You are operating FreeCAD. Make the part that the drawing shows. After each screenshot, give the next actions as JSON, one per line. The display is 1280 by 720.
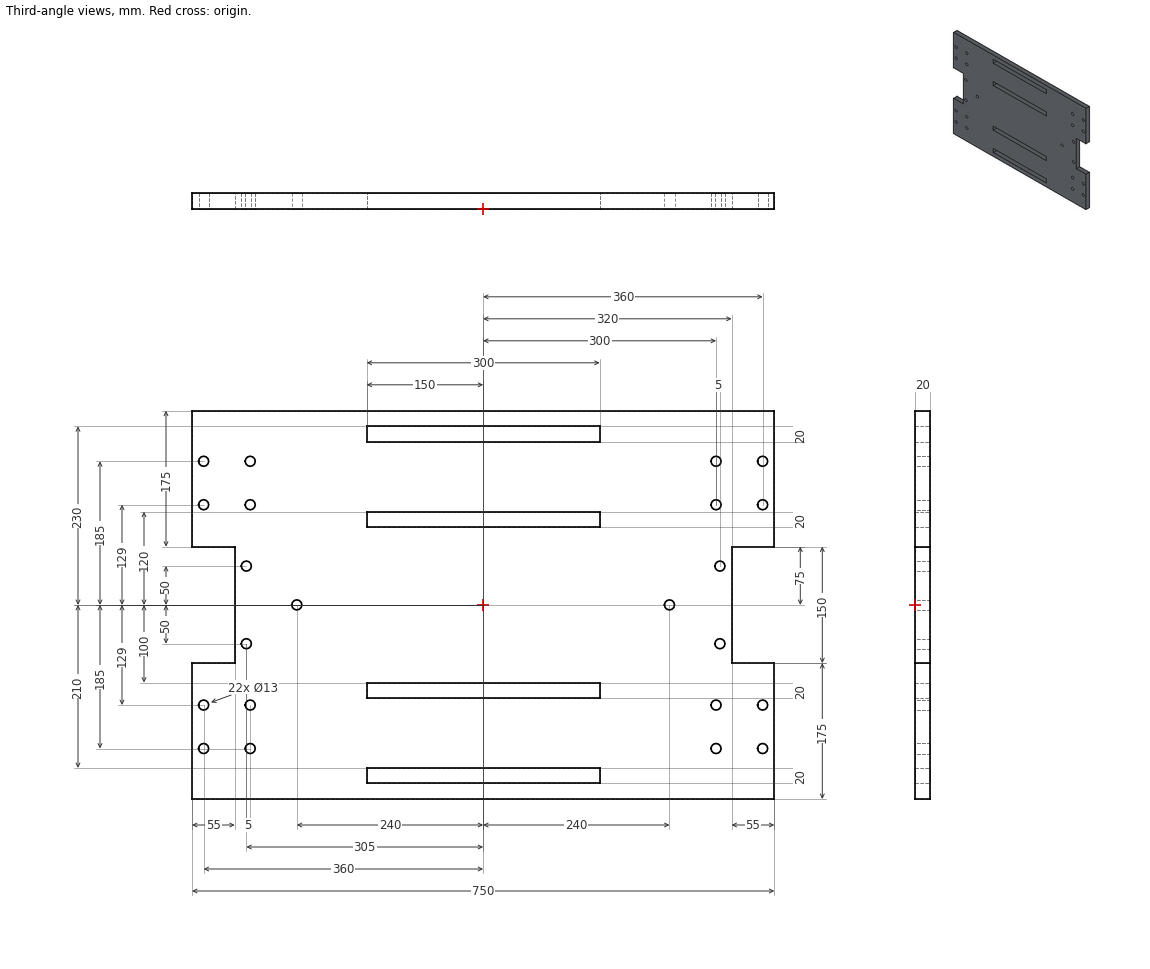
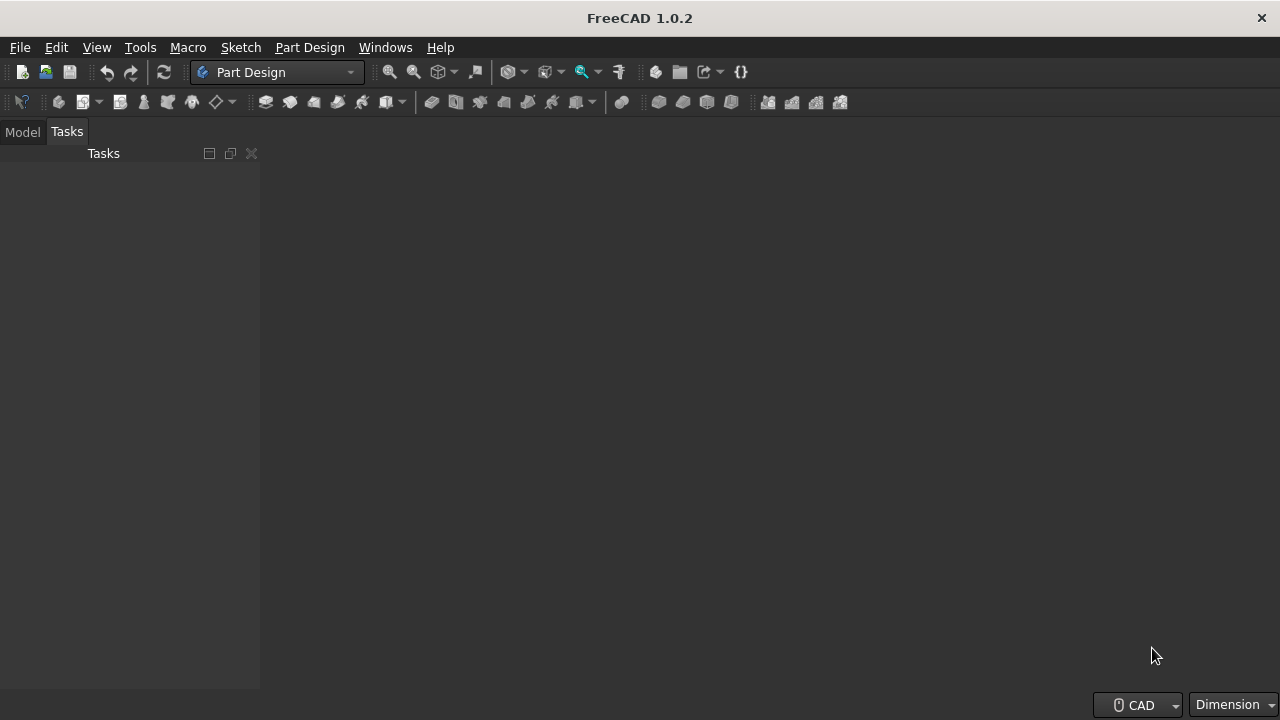
{"action": "left_click", "coordinate": [22, 72]}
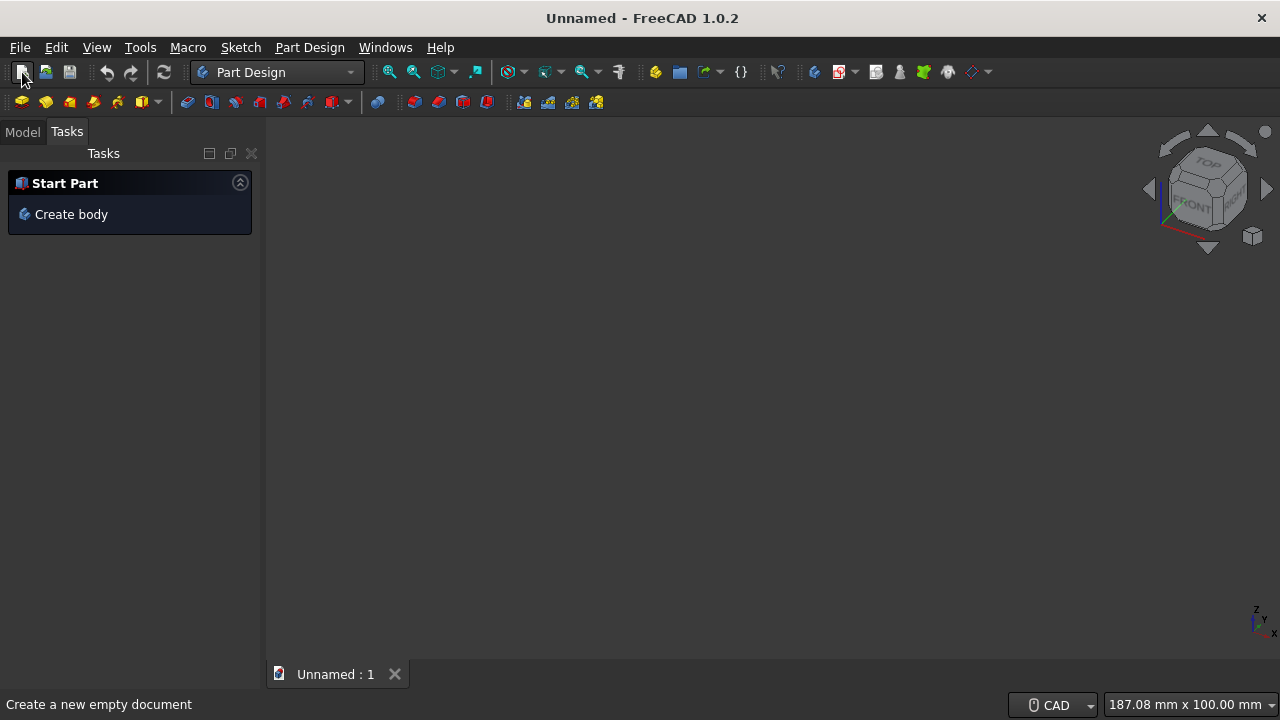
{"action": "left_click", "coordinate": [840, 72]}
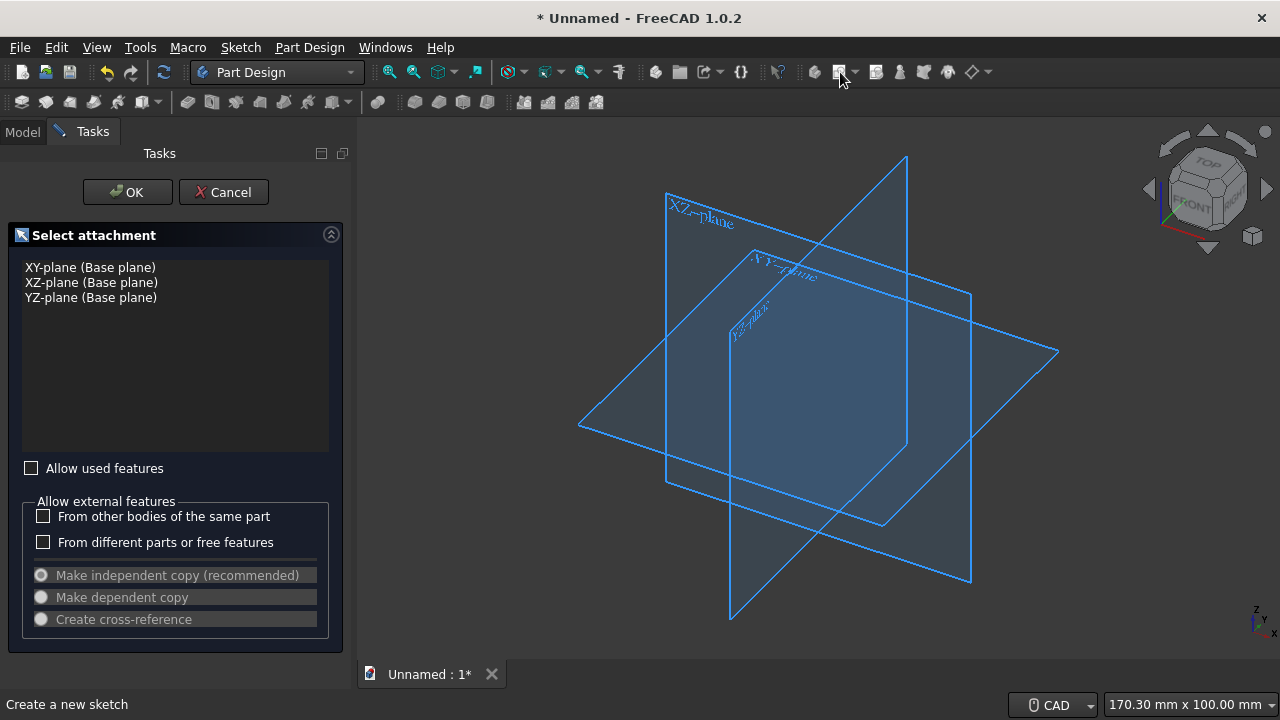
{"action": "left_click", "coordinate": [82, 282]}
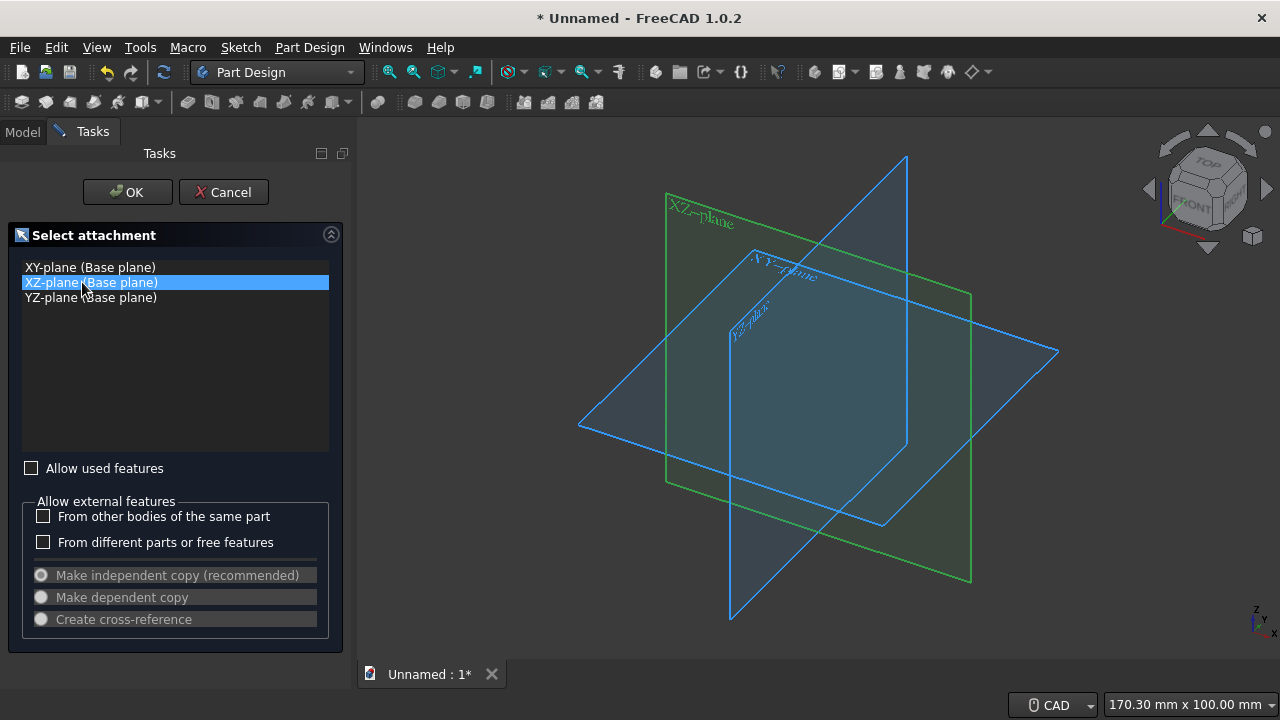
{"action": "left_click", "coordinate": [128, 192]}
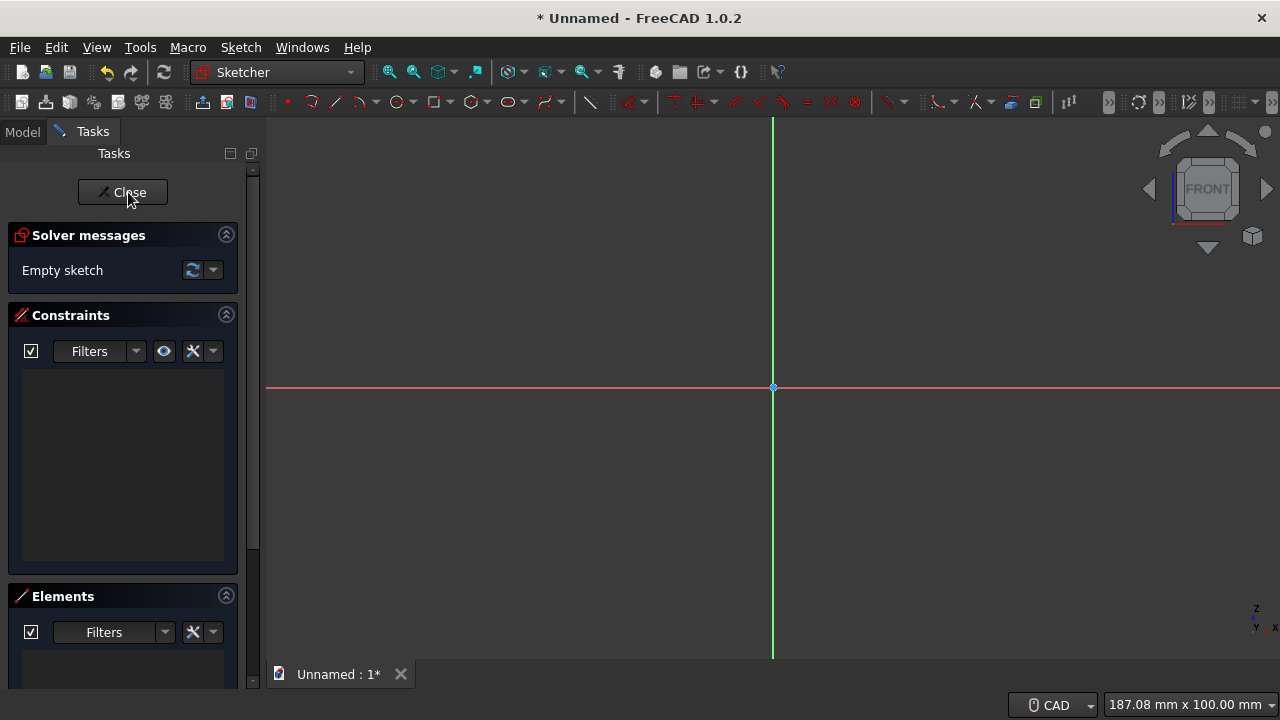
{"action": "scroll", "coordinate": [694, 388], "scroll_direction": "down", "scroll_amount": 10}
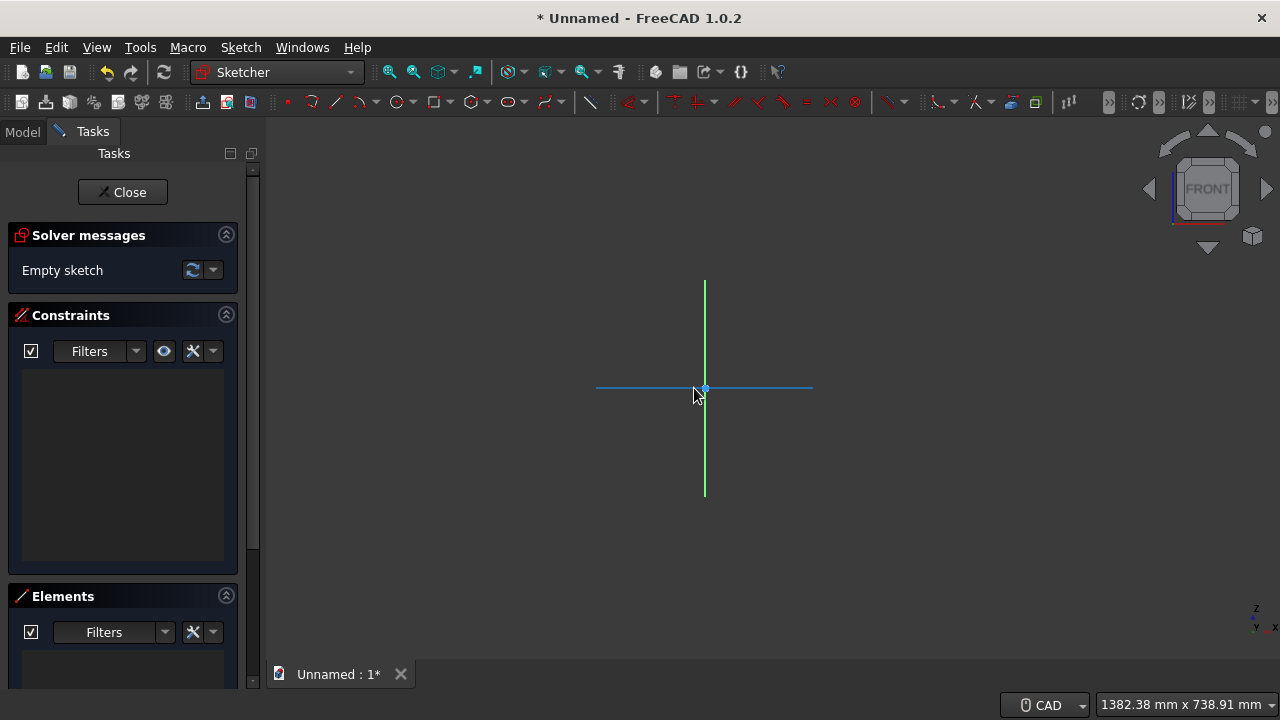
{"action": "left_click", "coordinate": [312, 102]}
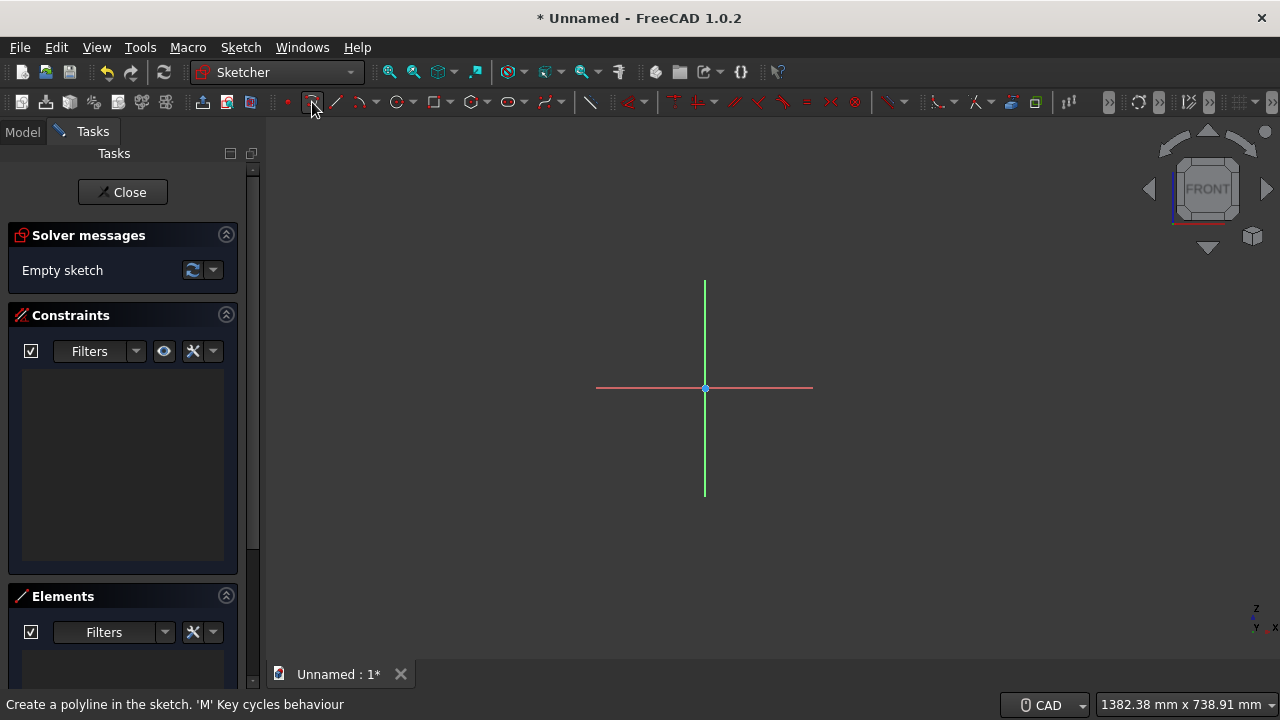
{"action": "left_click", "coordinate": [940, 333]}
{"action": "left_click", "coordinate": [940, 443]}
{"action": "left_click", "coordinate": [980, 443]}
{"action": "left_click", "coordinate": [980, 572]}
{"action": "left_click", "coordinate": [430, 572]}
{"action": "left_click", "coordinate": [430, 443]}
{"action": "left_click", "coordinate": [470, 443]}
{"action": "left_click", "coordinate": [470, 333]}
{"action": "left_click", "coordinate": [430, 333]}
{"action": "left_click", "coordinate": [430, 205]}
{"action": "left_click", "coordinate": [980, 205]}
{"action": "left_click", "coordinate": [980, 333]}
{"action": "left_click", "coordinate": [940, 334]}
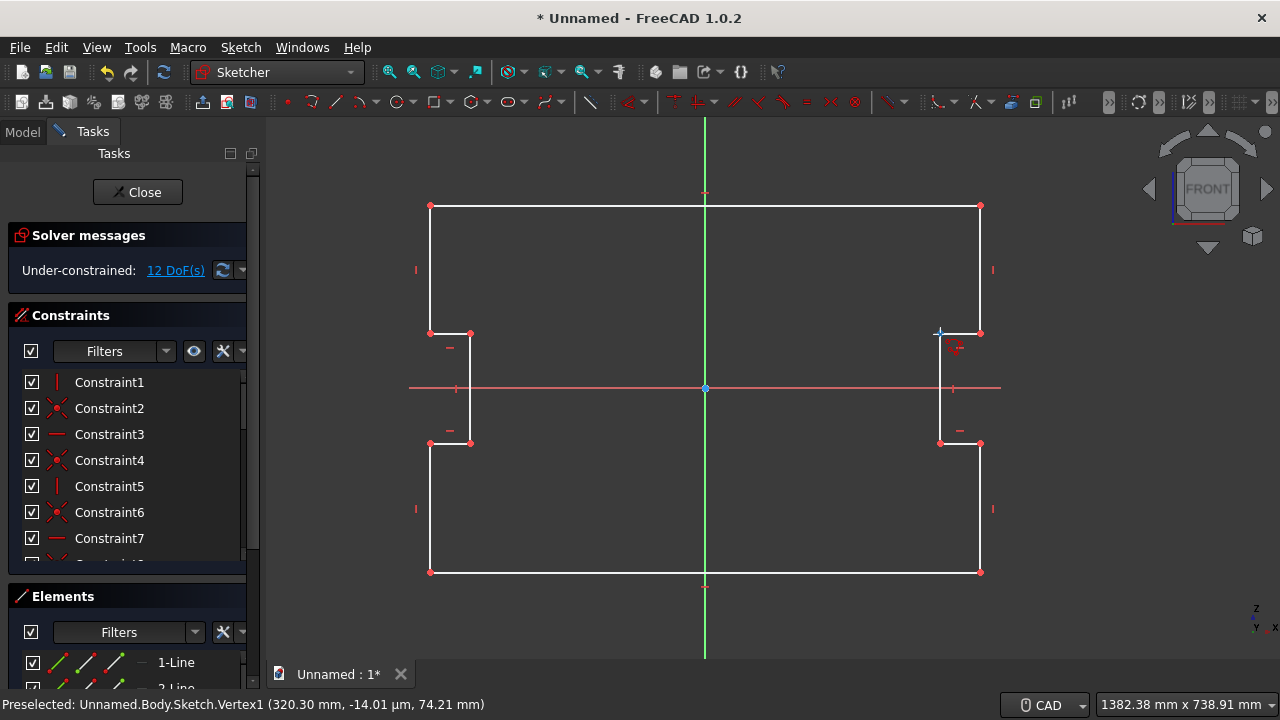
{"action": "left_click", "coordinate": [434, 102]}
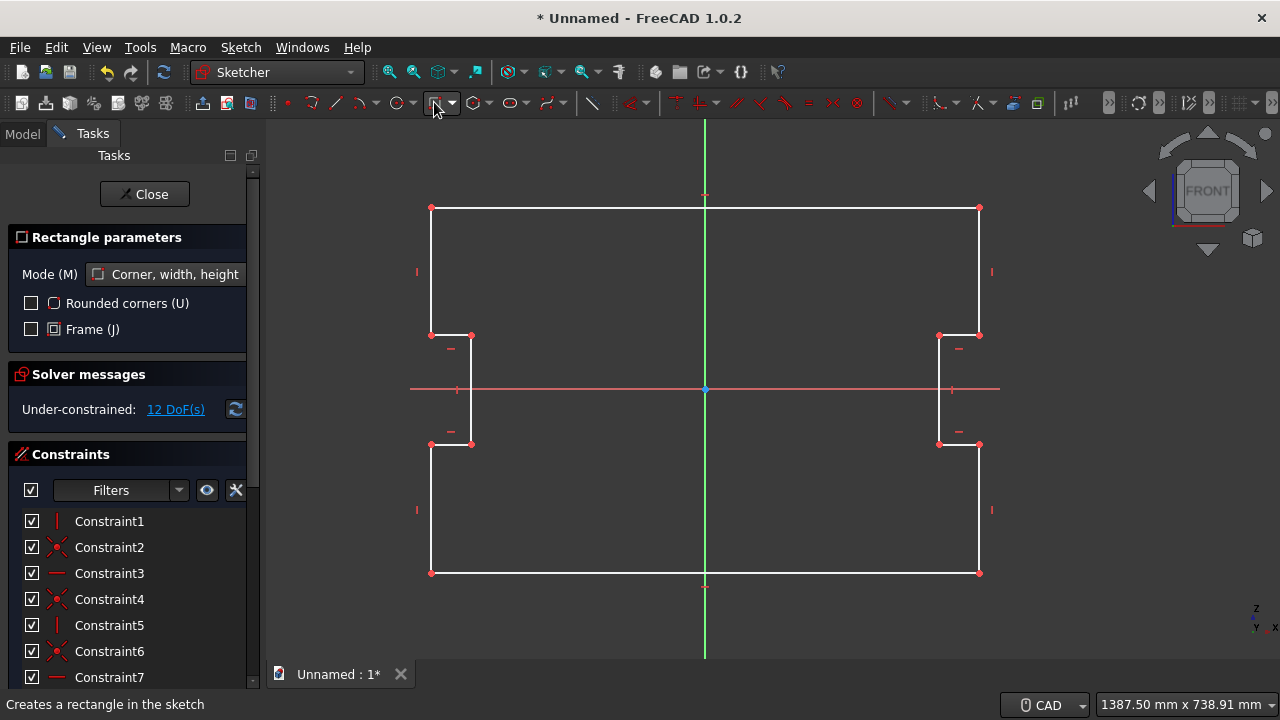
{"action": "left_click", "coordinate": [596, 221]}
{"action": "mouse_move", "coordinate": [815, 236]}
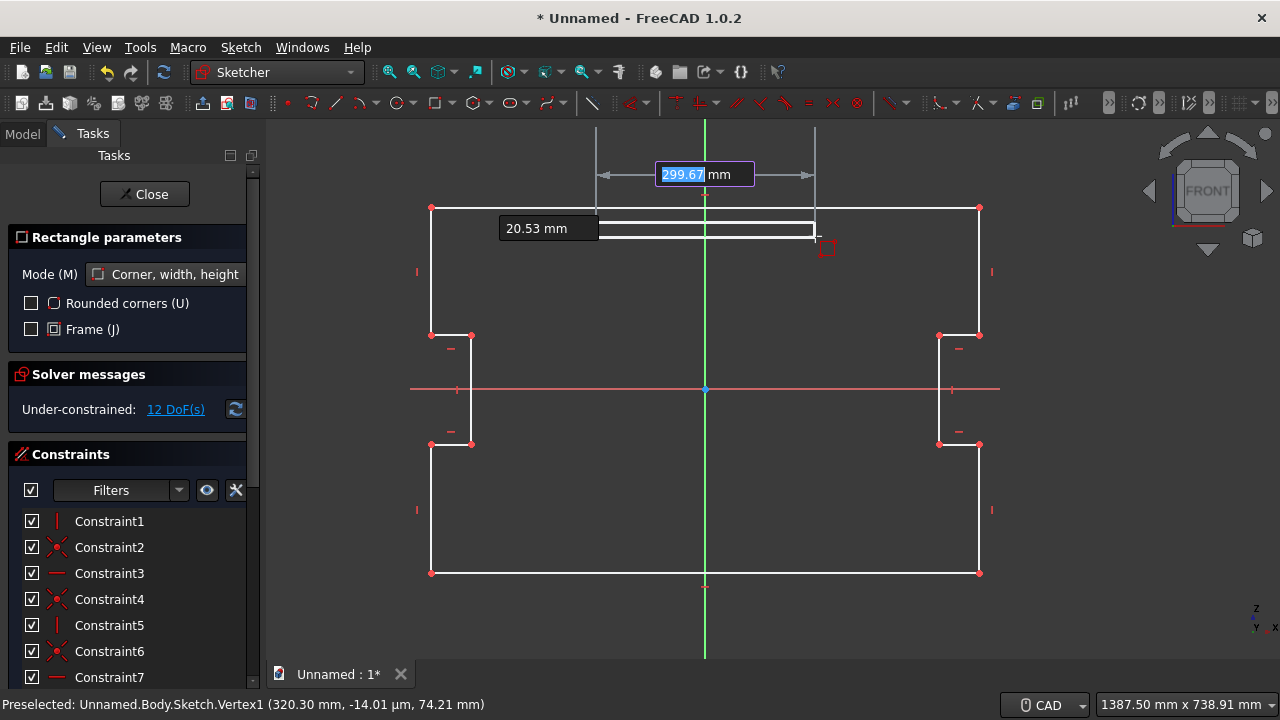
{"action": "type", "text": "300"}
{"action": "key", "text": "Tab"}
{"action": "type", "text": "20"}
{"action": "key", "text": "Return"}